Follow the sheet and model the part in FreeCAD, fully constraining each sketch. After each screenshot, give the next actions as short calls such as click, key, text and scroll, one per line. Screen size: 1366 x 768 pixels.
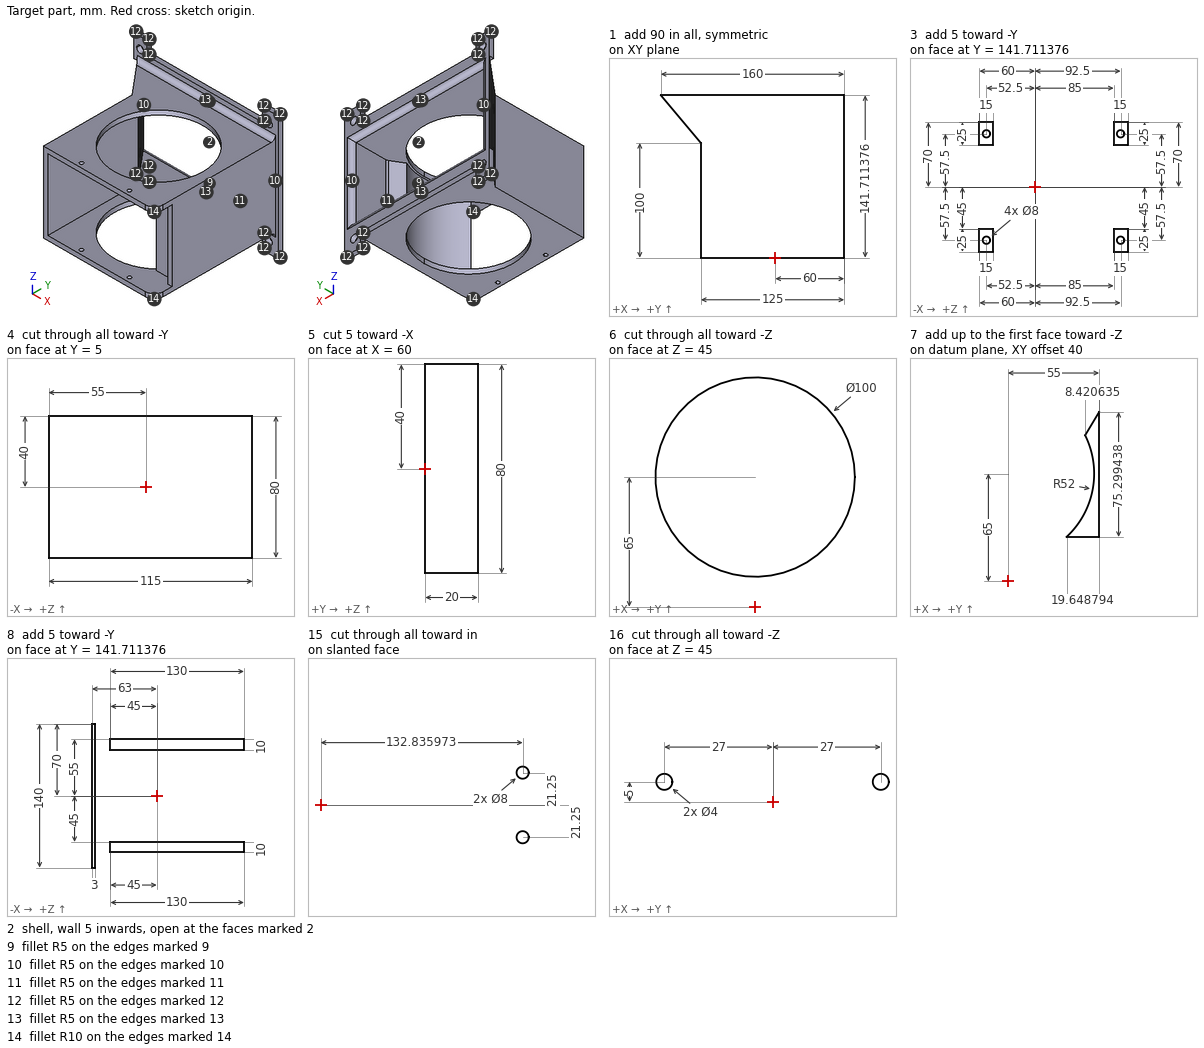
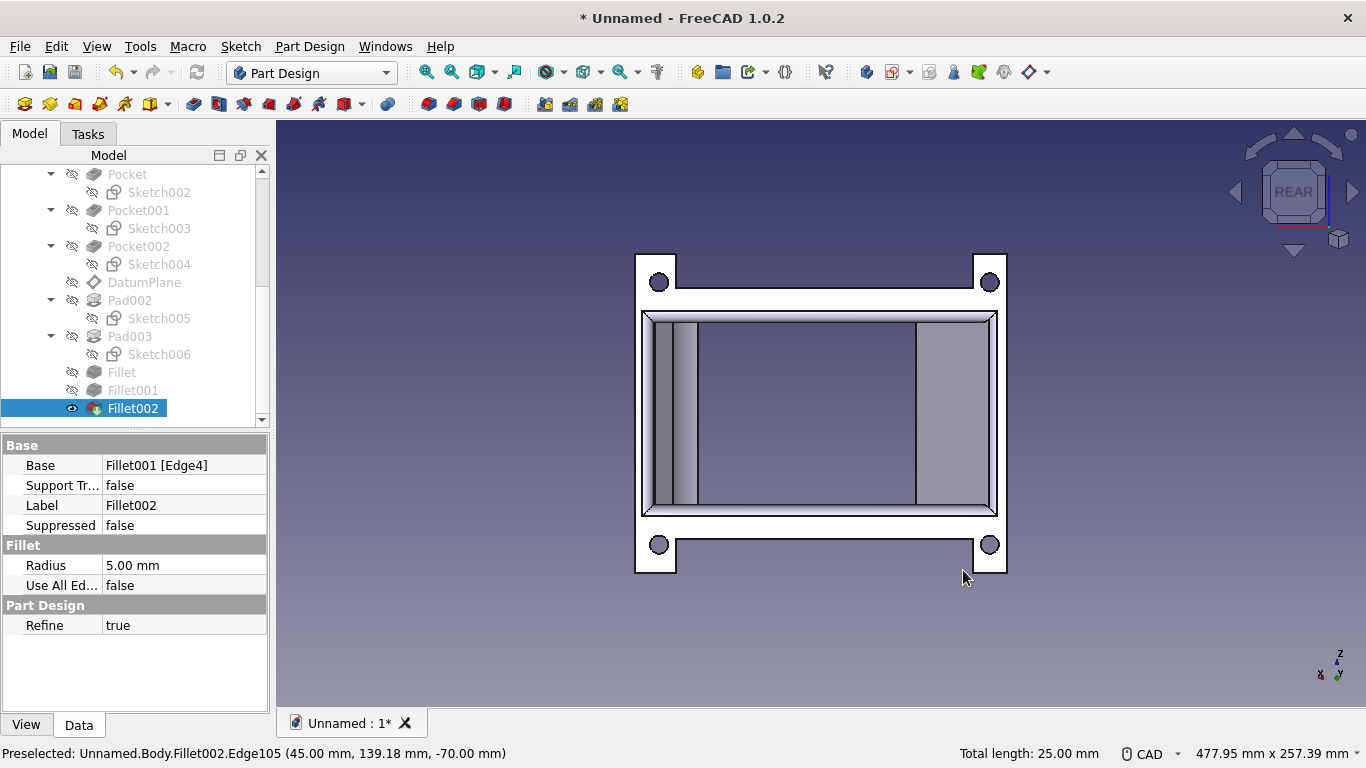
scroll(676, 538, up, 7)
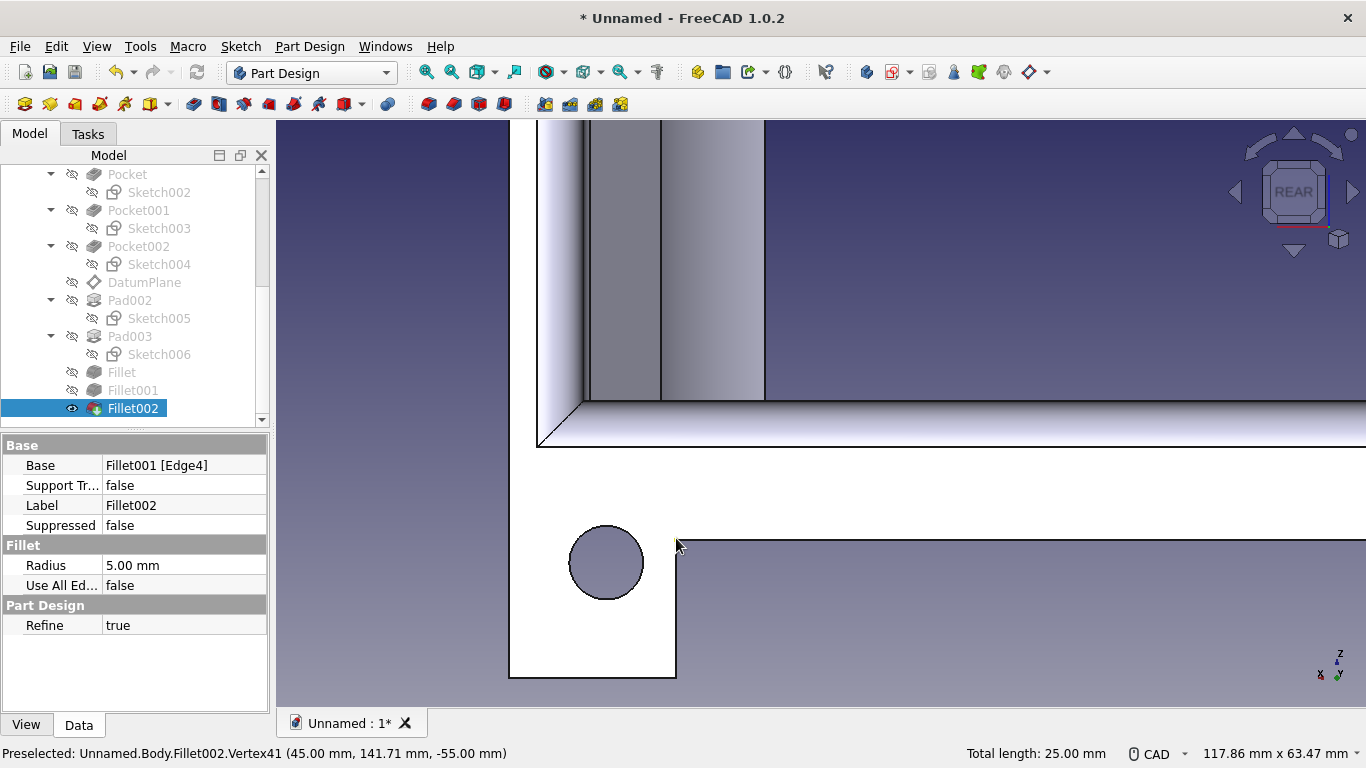
click(427, 72)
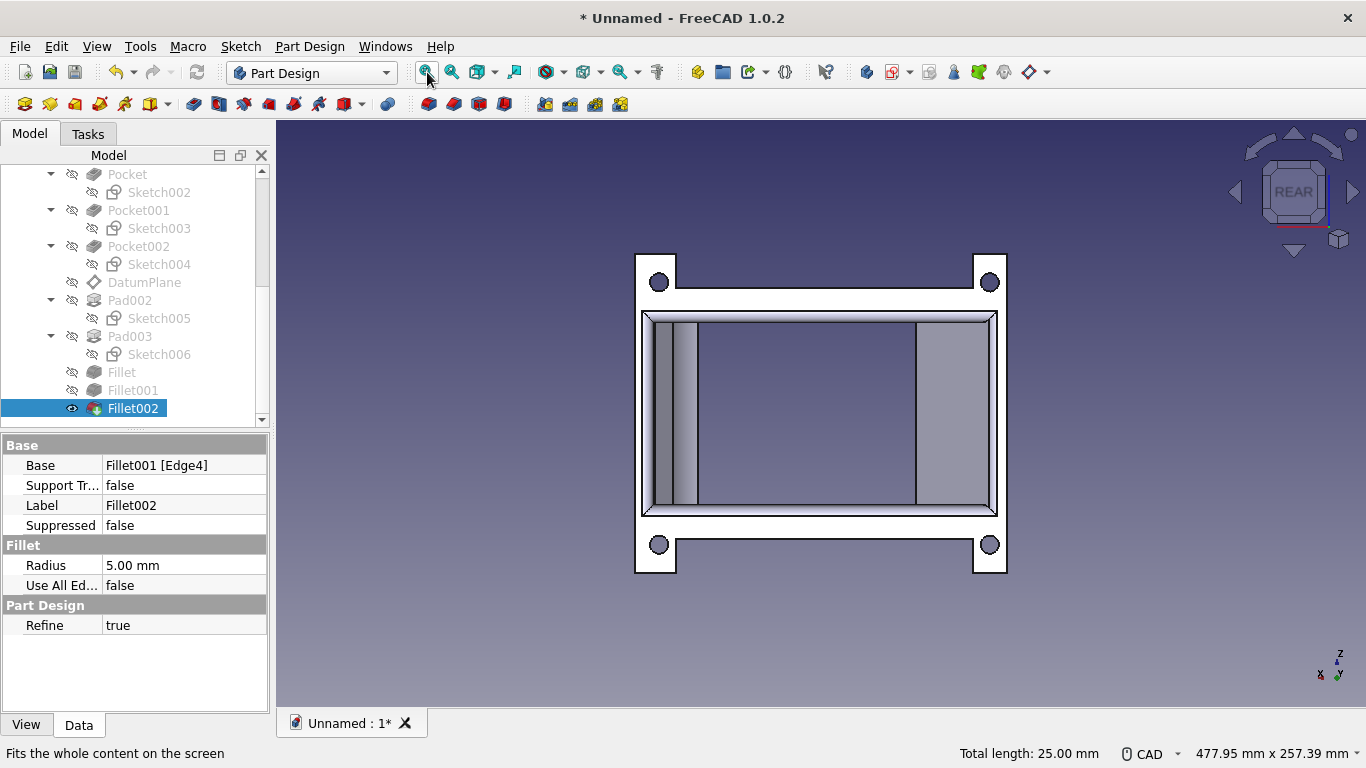
key(6)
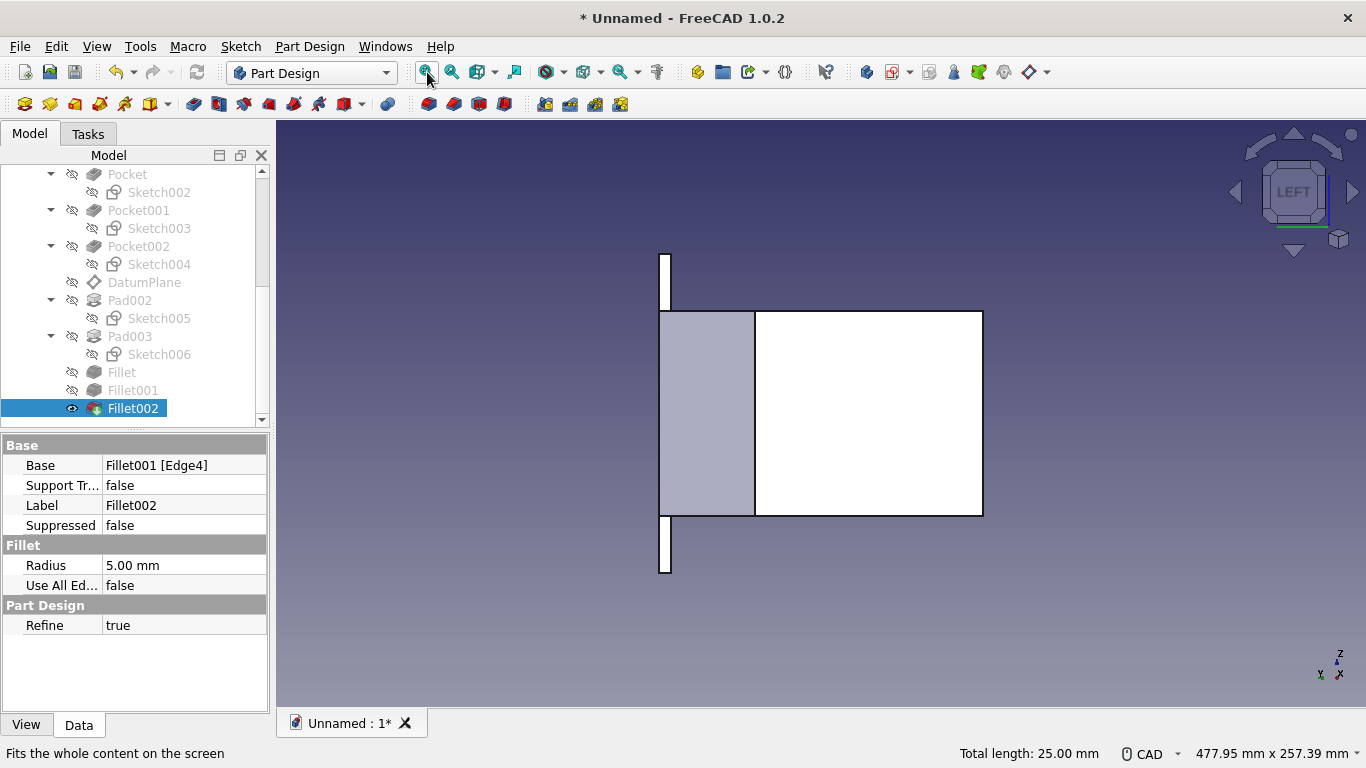
scroll(665, 538, up, 7)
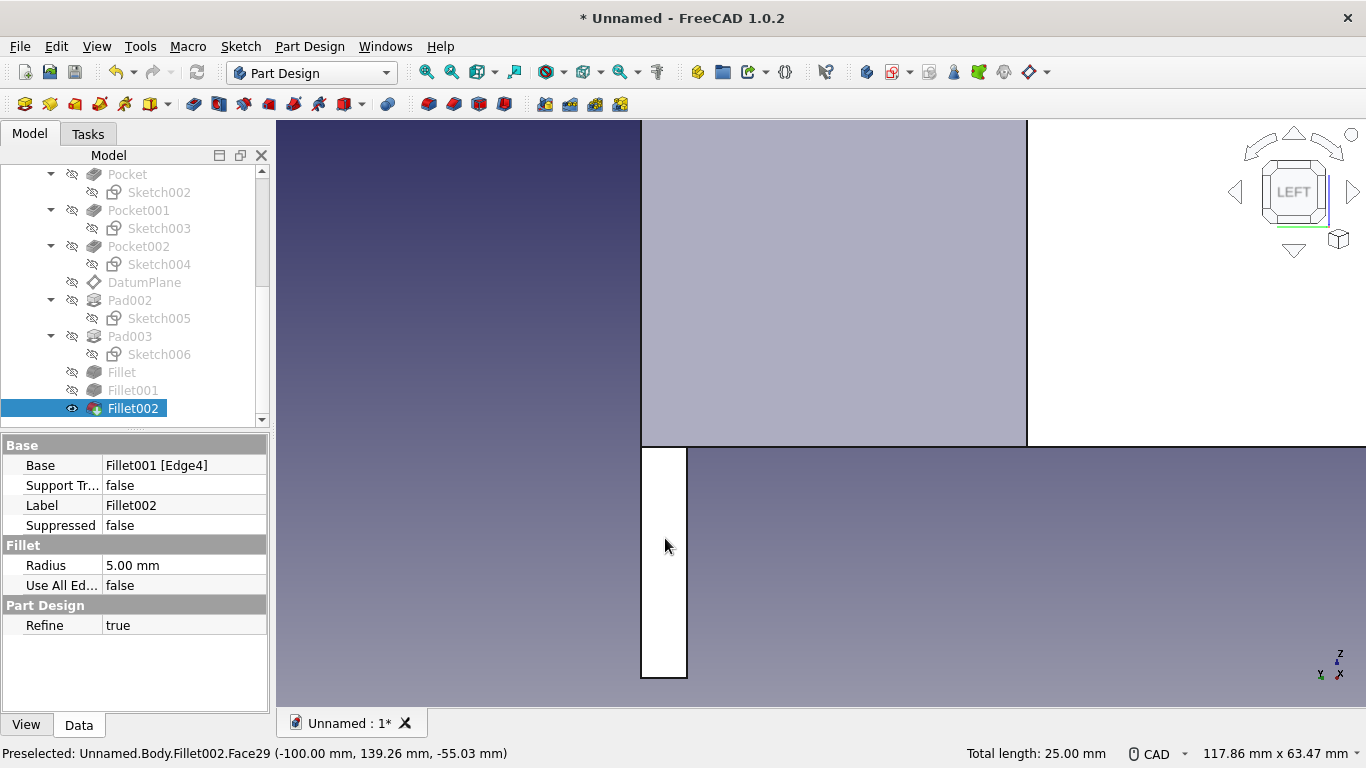
click(664, 677, ctrl)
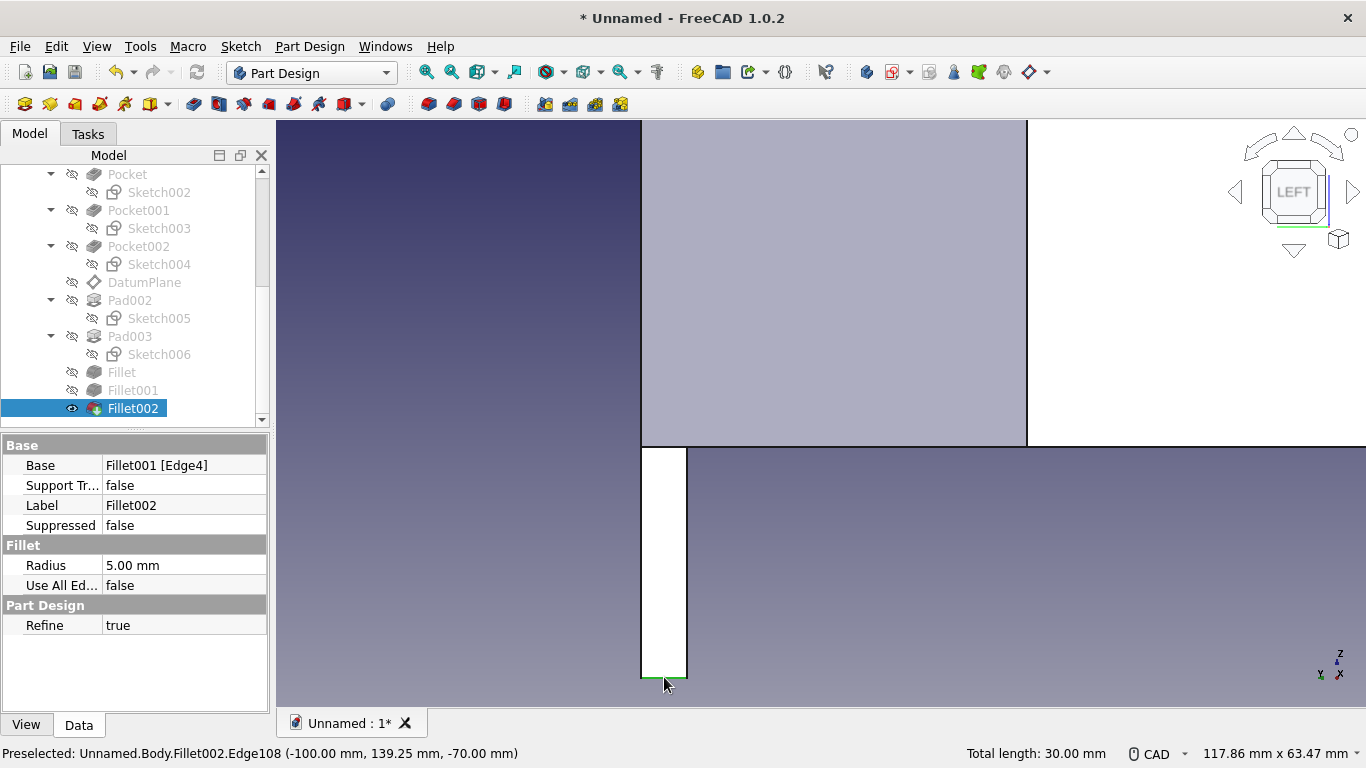
key(v)
key(f)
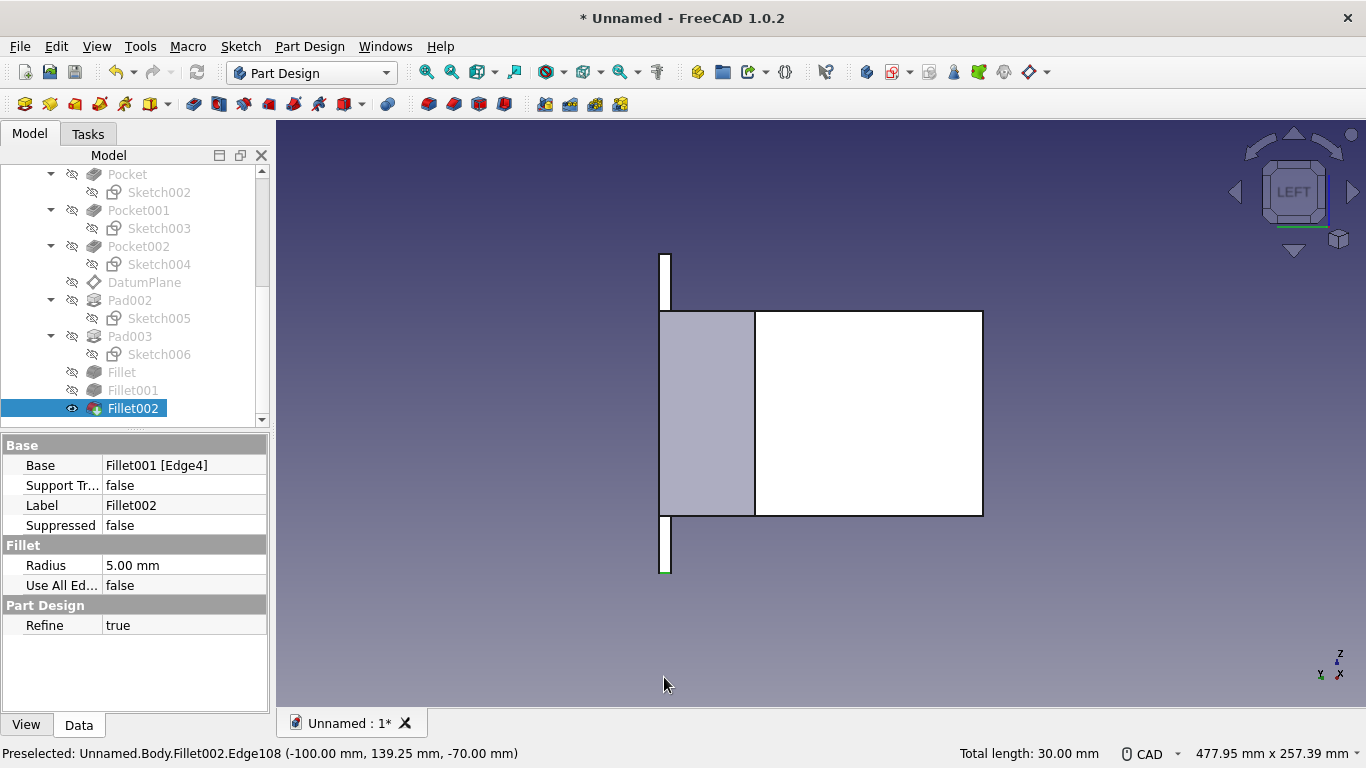
key(v)
key(3)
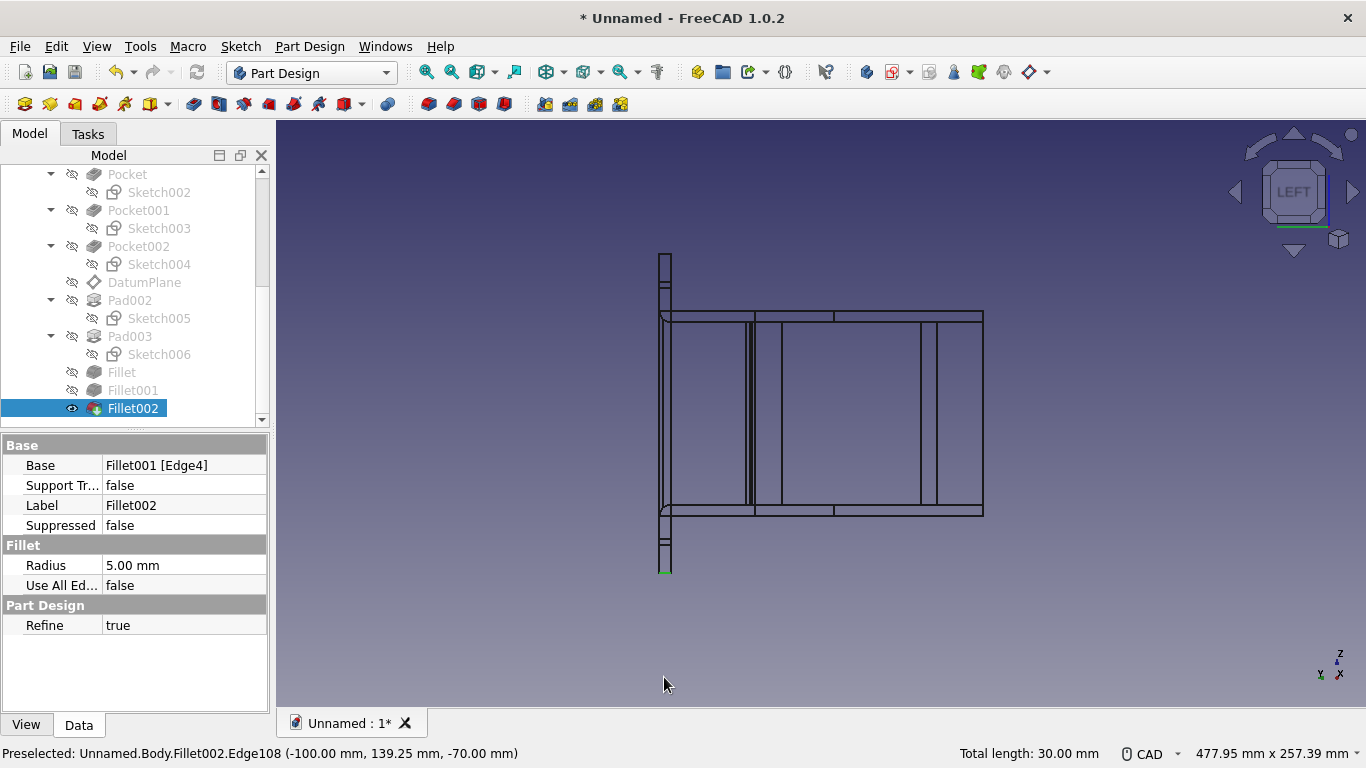
key(0)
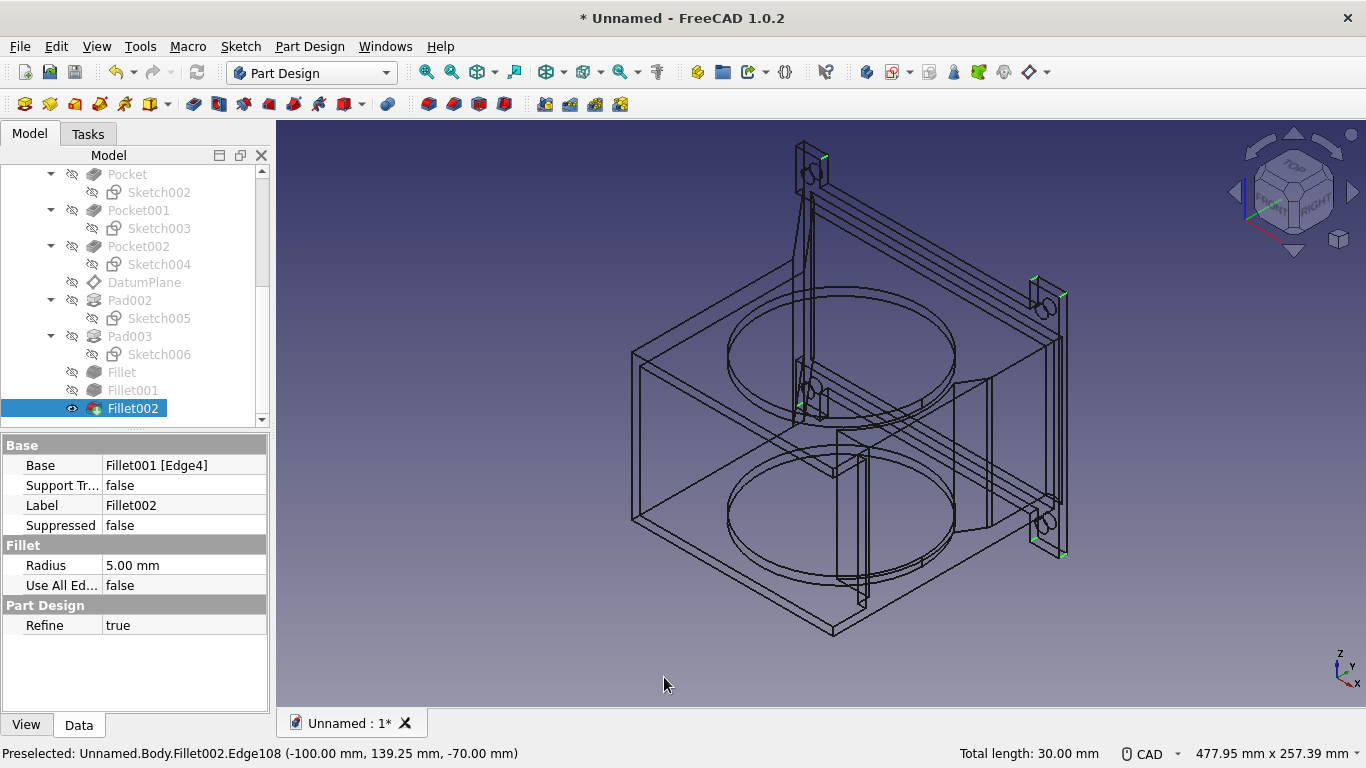
click(1035, 509, ctrl)